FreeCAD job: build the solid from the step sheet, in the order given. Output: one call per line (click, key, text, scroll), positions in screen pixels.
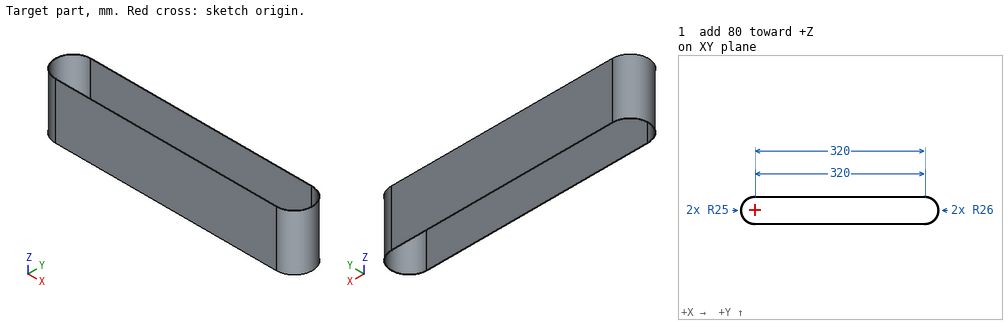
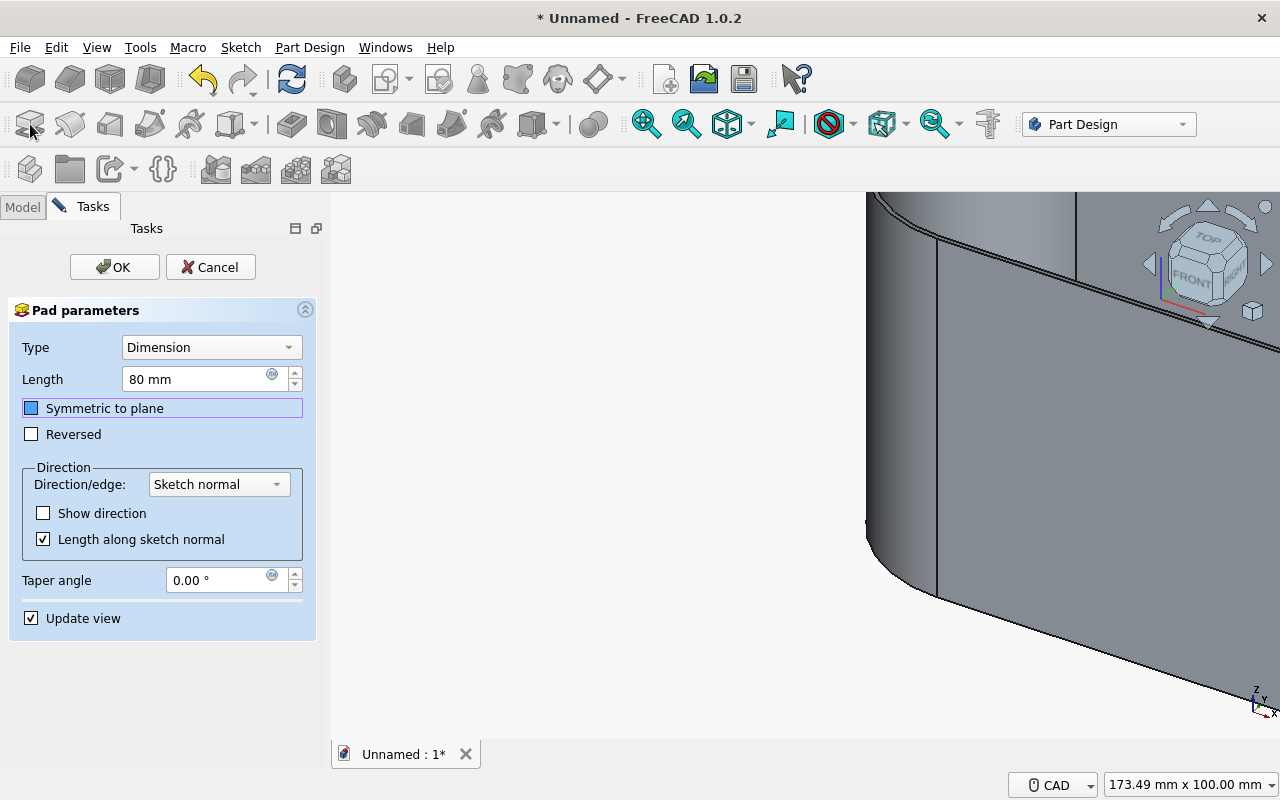
click(115, 267)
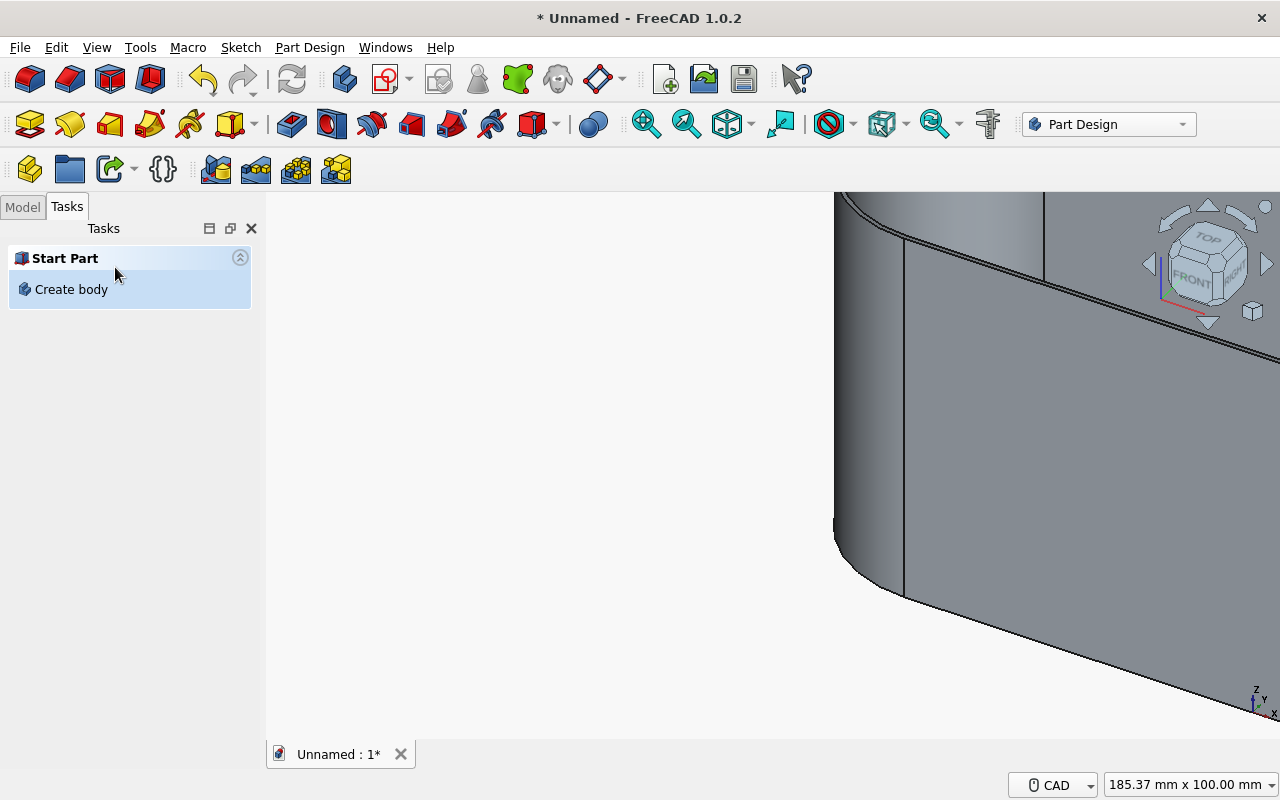
key(0)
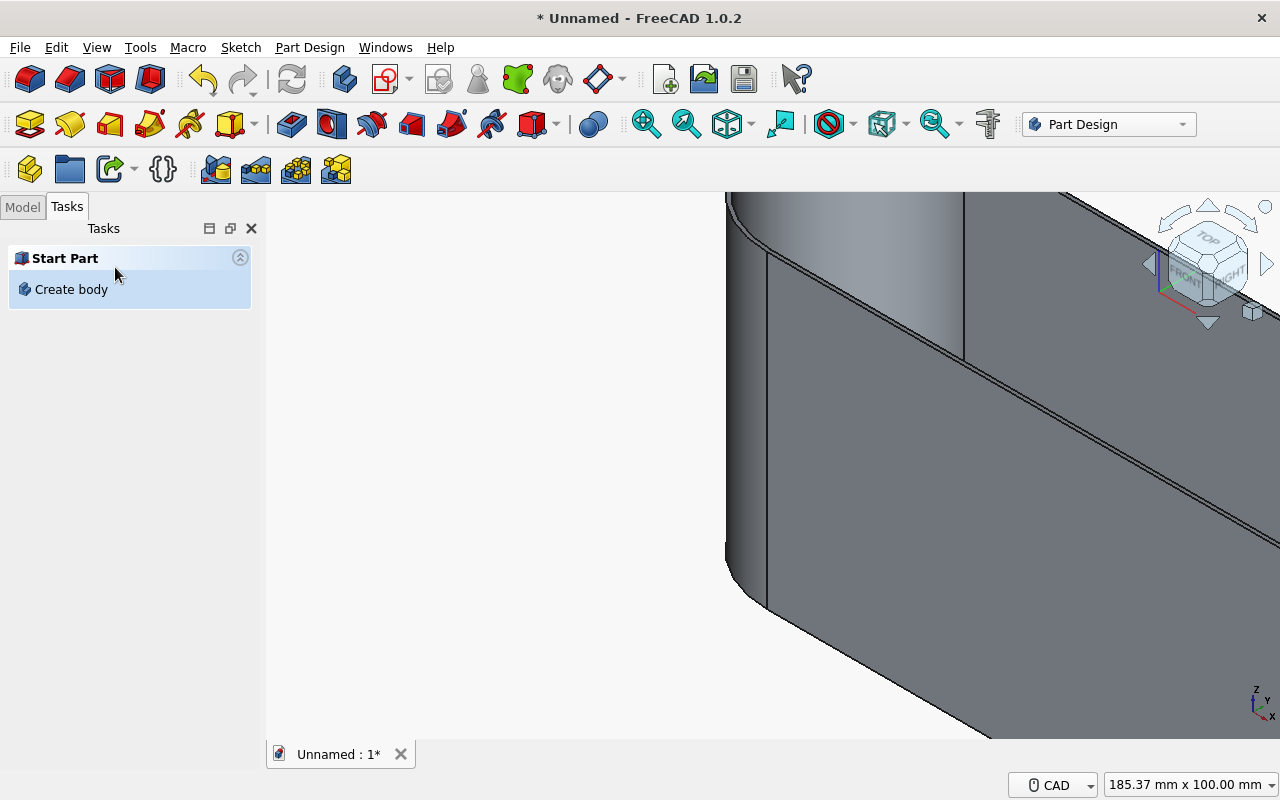
click(648, 124)